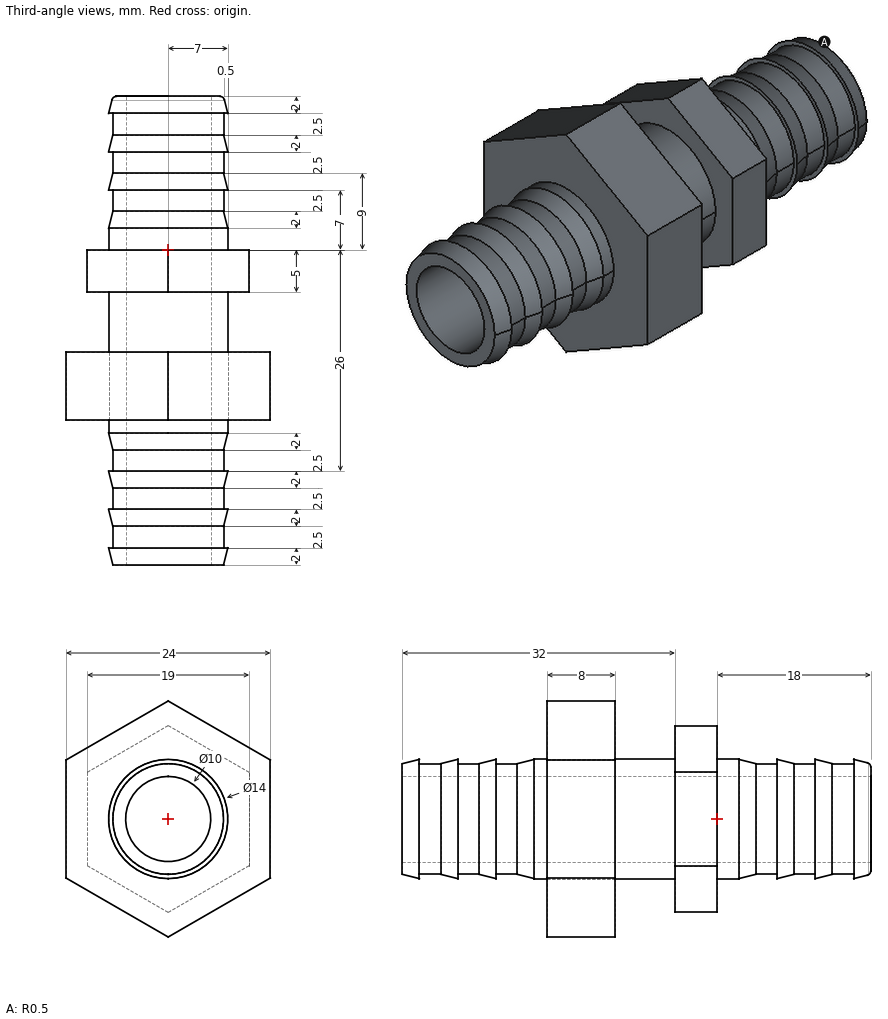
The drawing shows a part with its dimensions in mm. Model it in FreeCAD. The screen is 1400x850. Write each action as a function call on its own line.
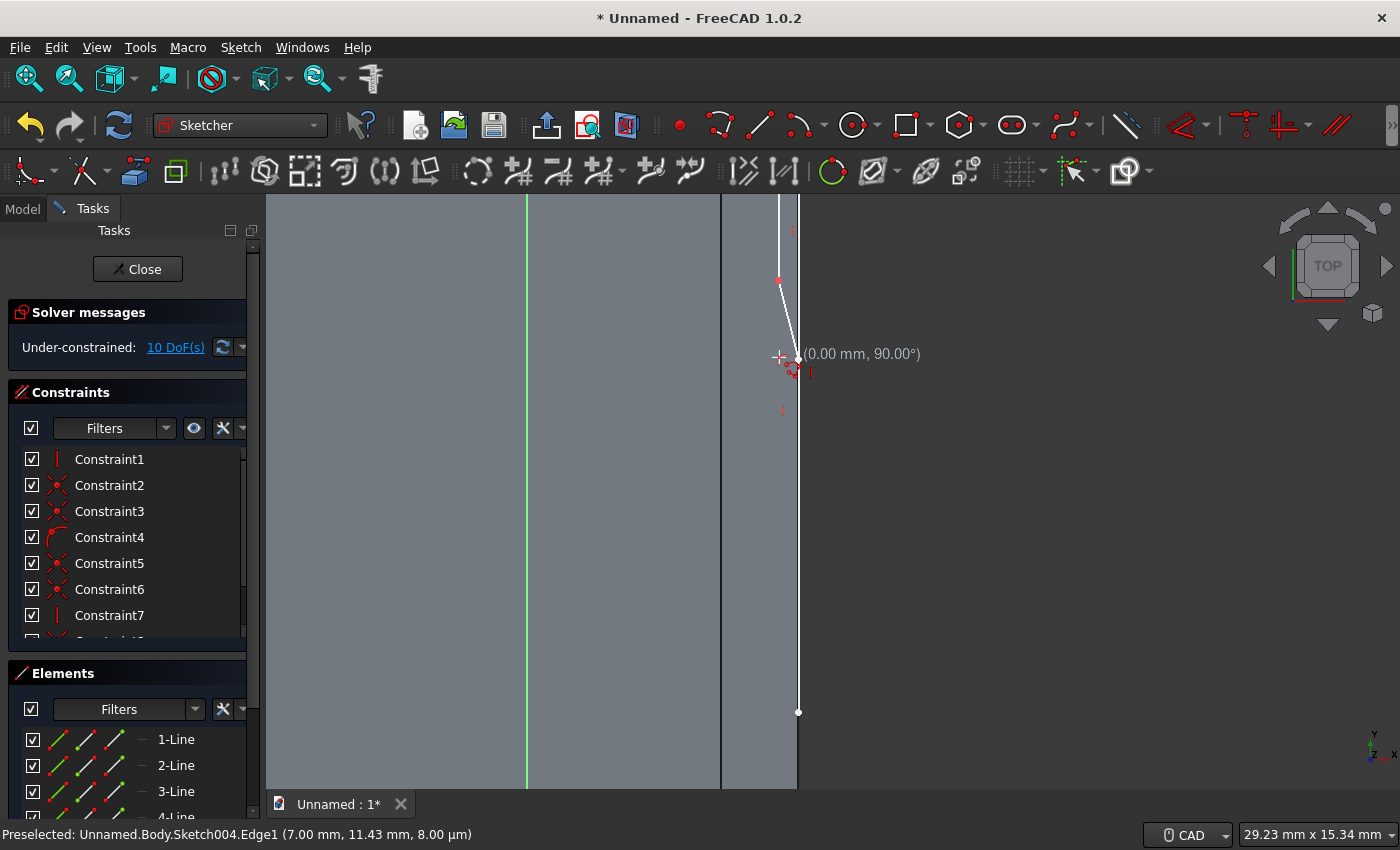
click(779, 357)
click(779, 454)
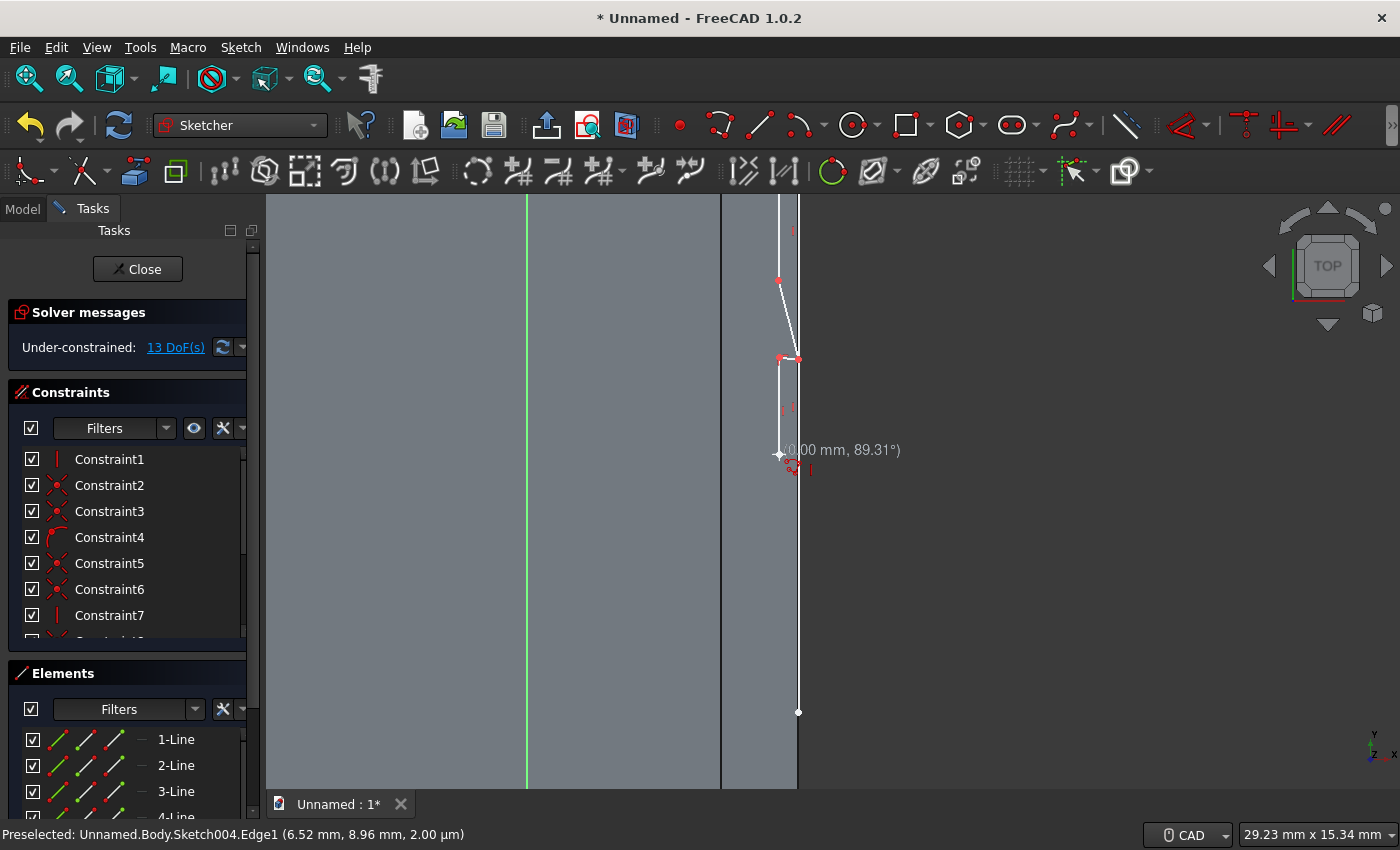
scroll(785, 357, down, 9)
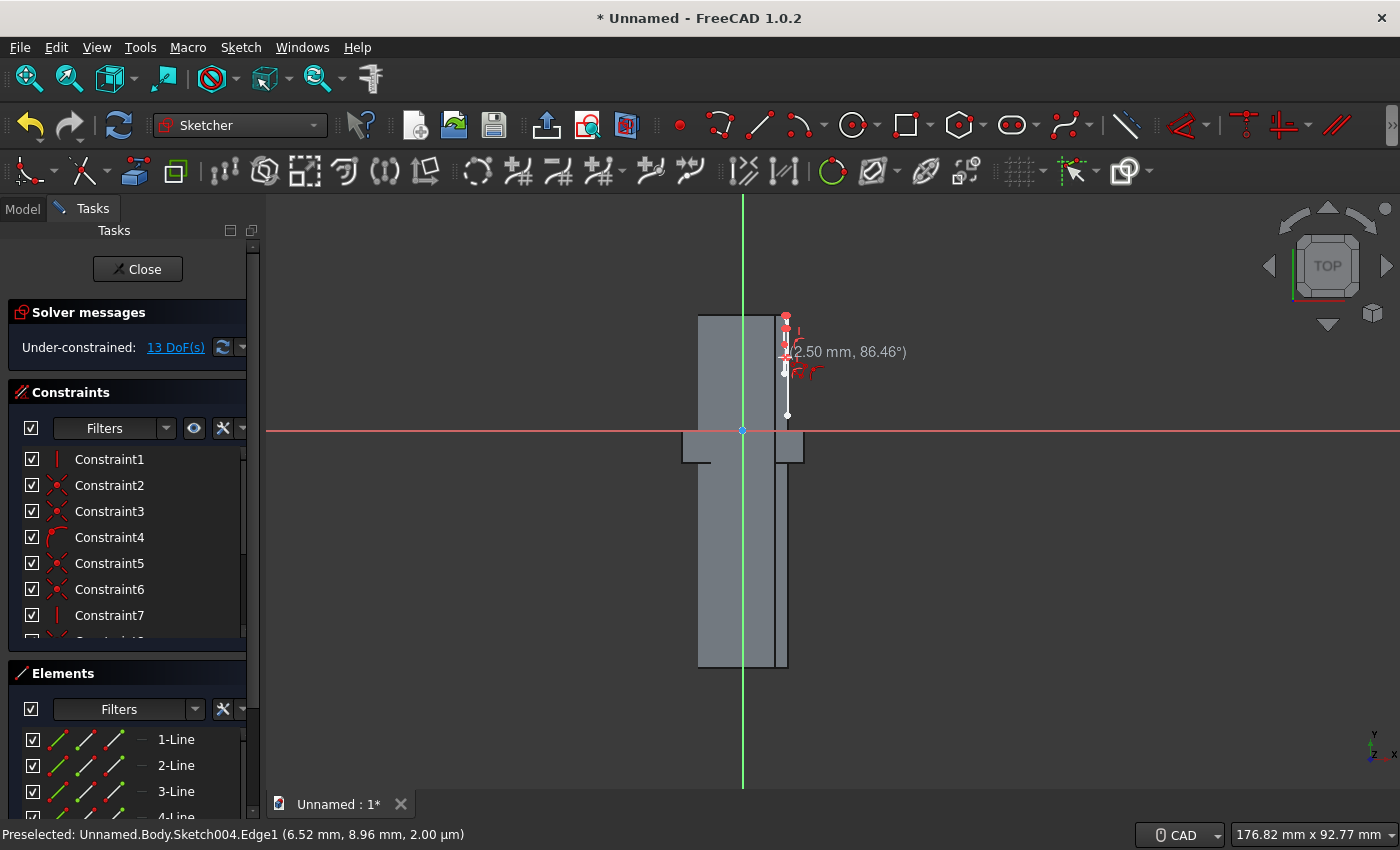
click(788, 386)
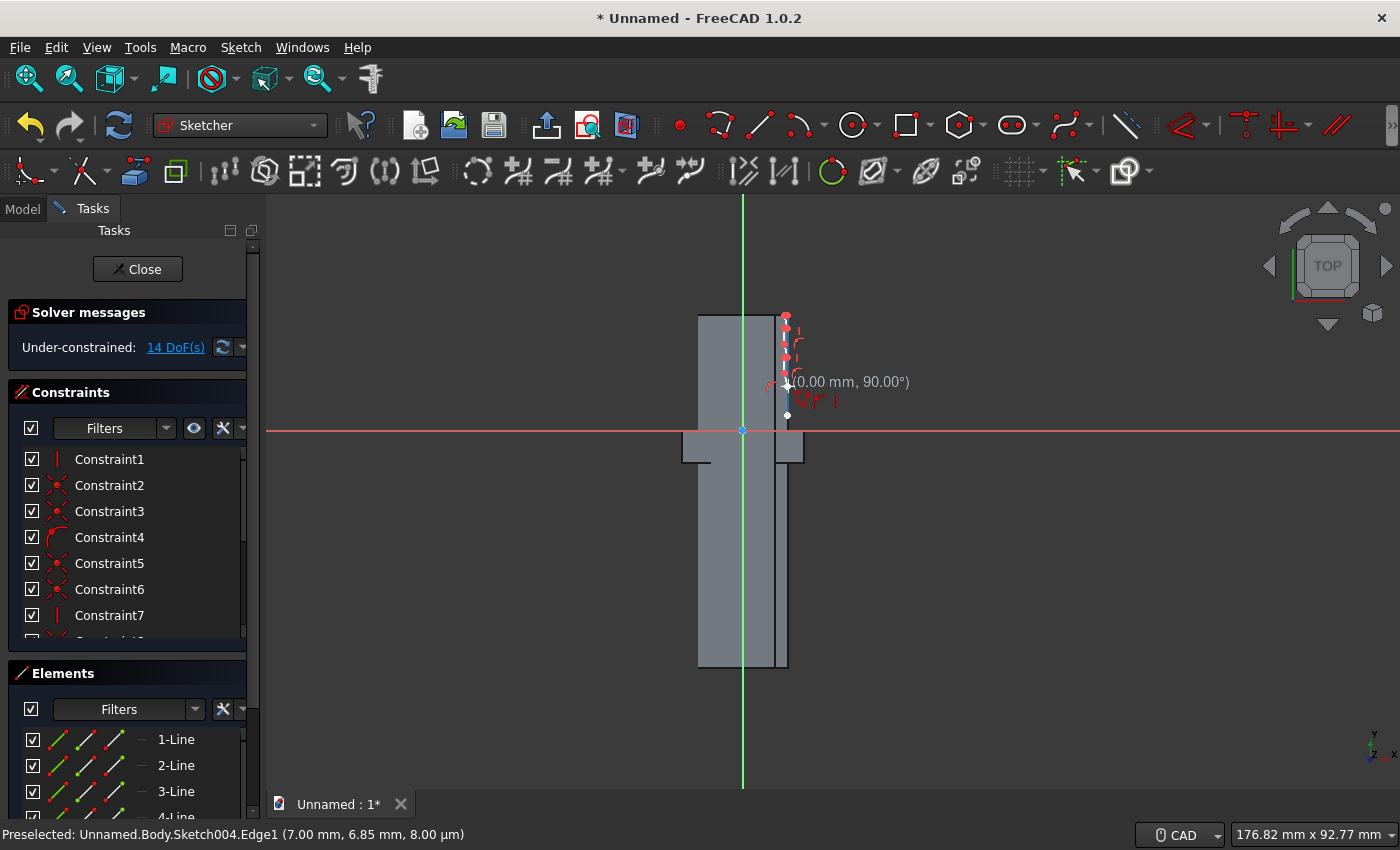
scroll(784, 386, up, 9)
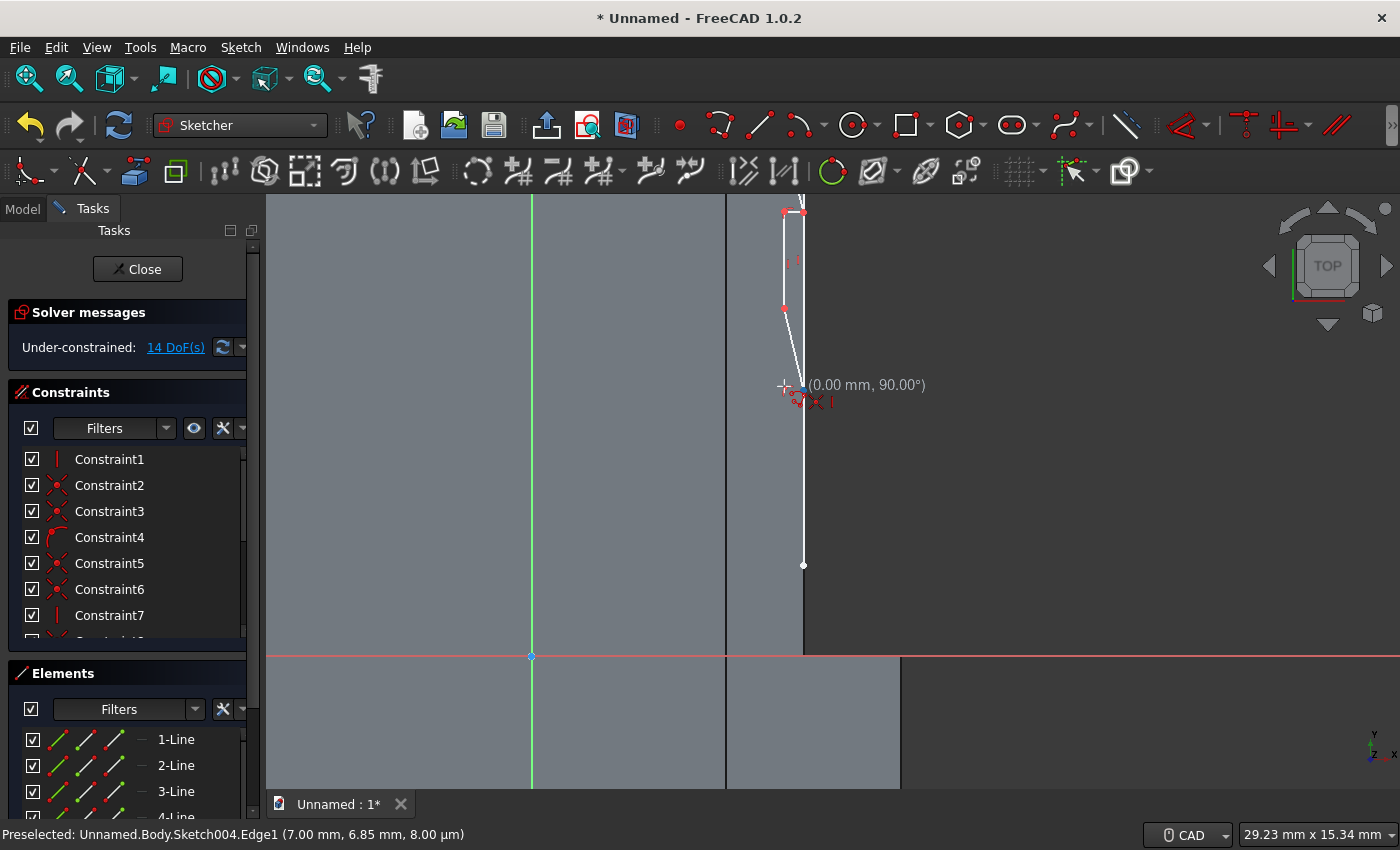
click(784, 384)
click(784, 481)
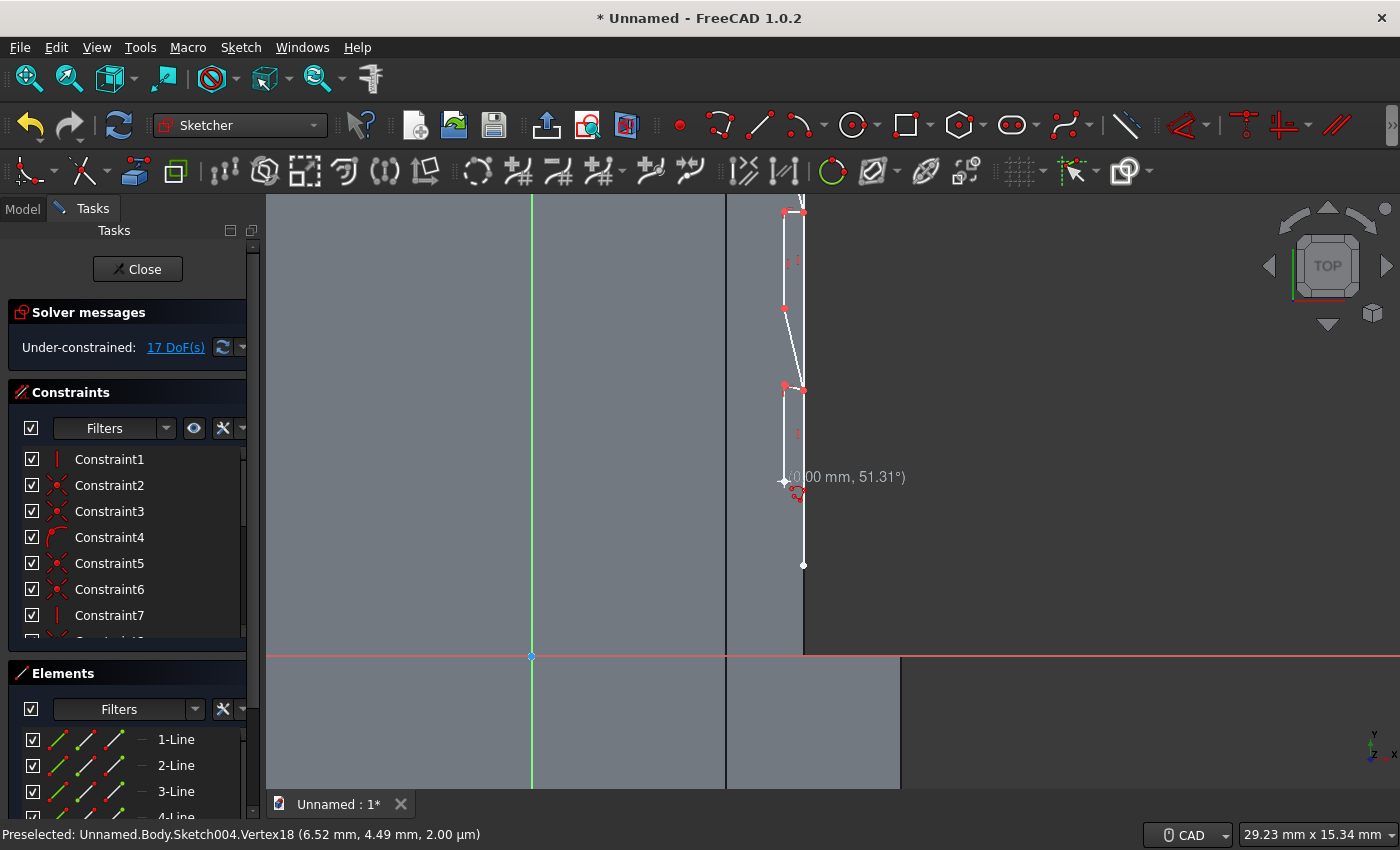
scroll(784, 386, down, 9)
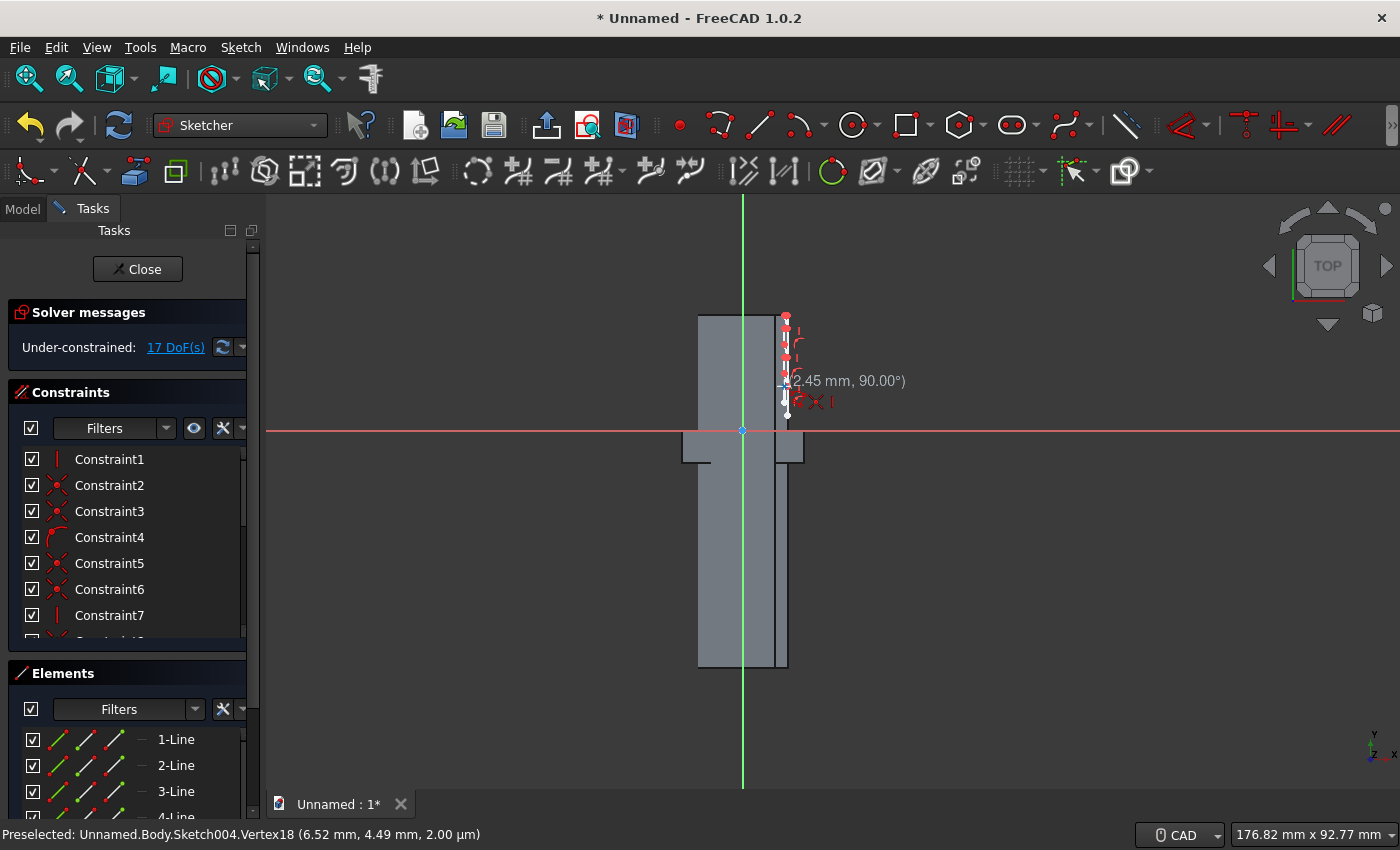
click(788, 416)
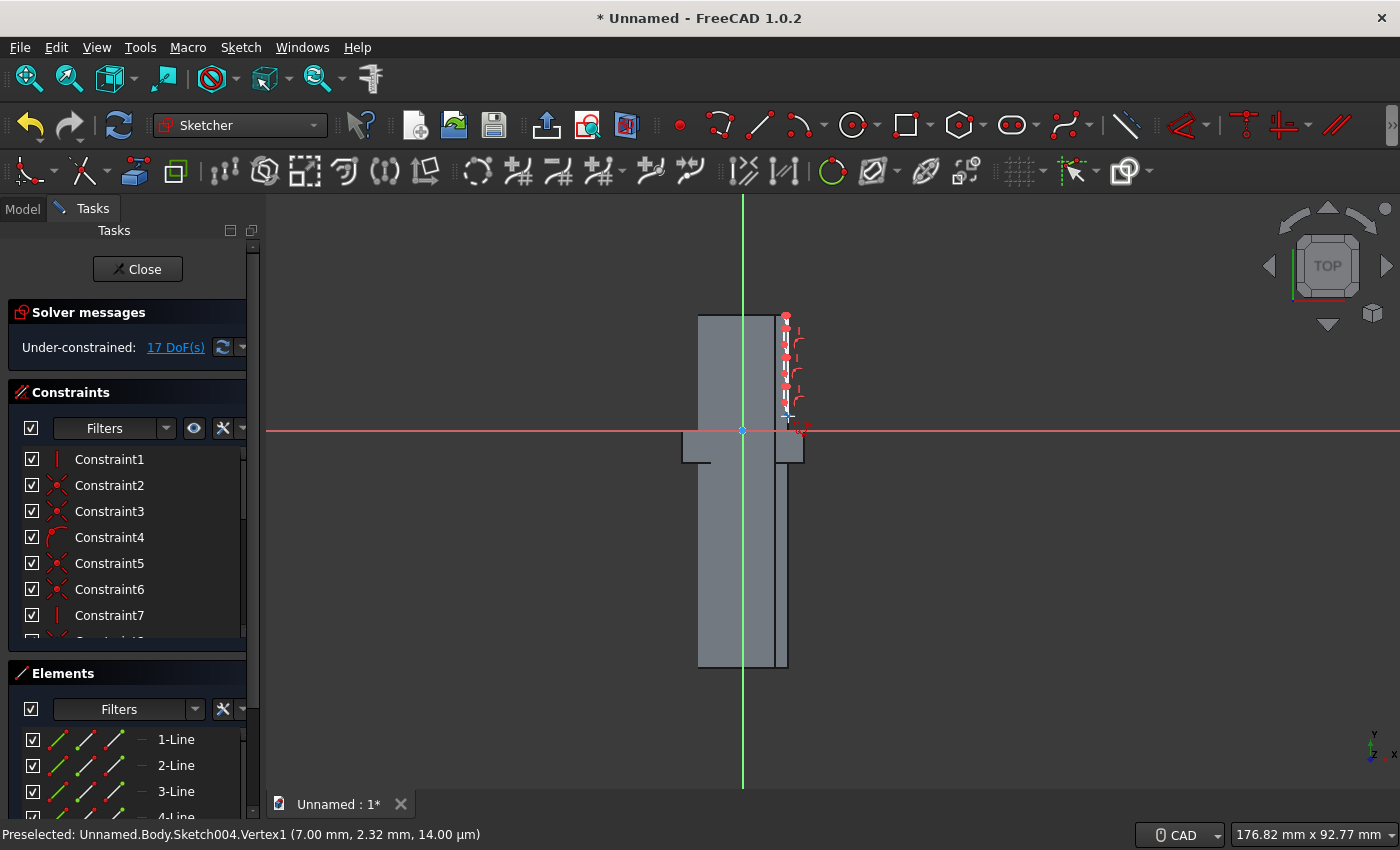
click(788, 569)
click(784, 582)
click(784, 598)